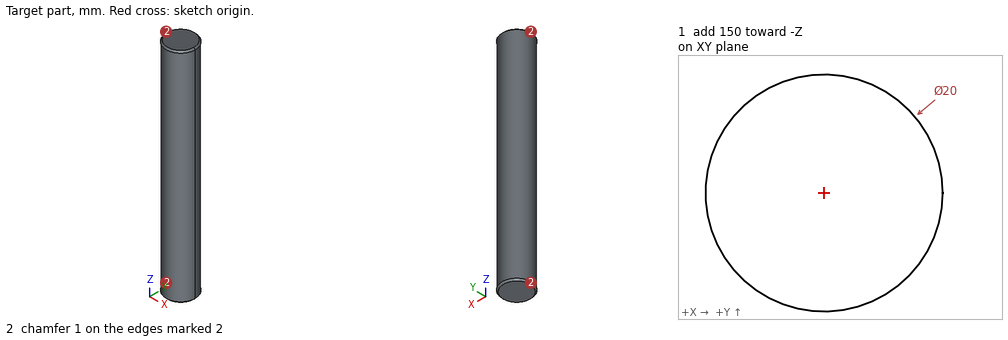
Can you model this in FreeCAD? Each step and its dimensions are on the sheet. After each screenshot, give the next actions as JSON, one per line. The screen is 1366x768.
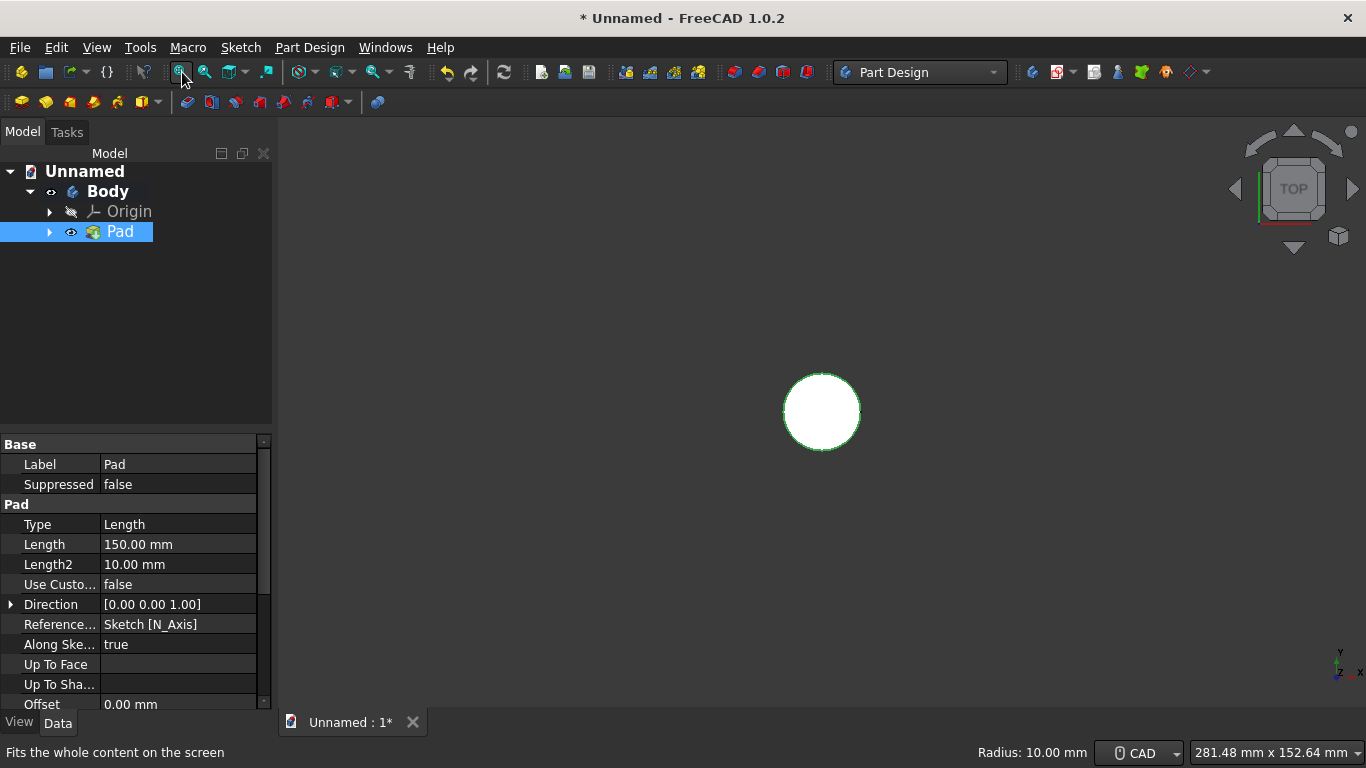
{"action": "key", "text": "1"}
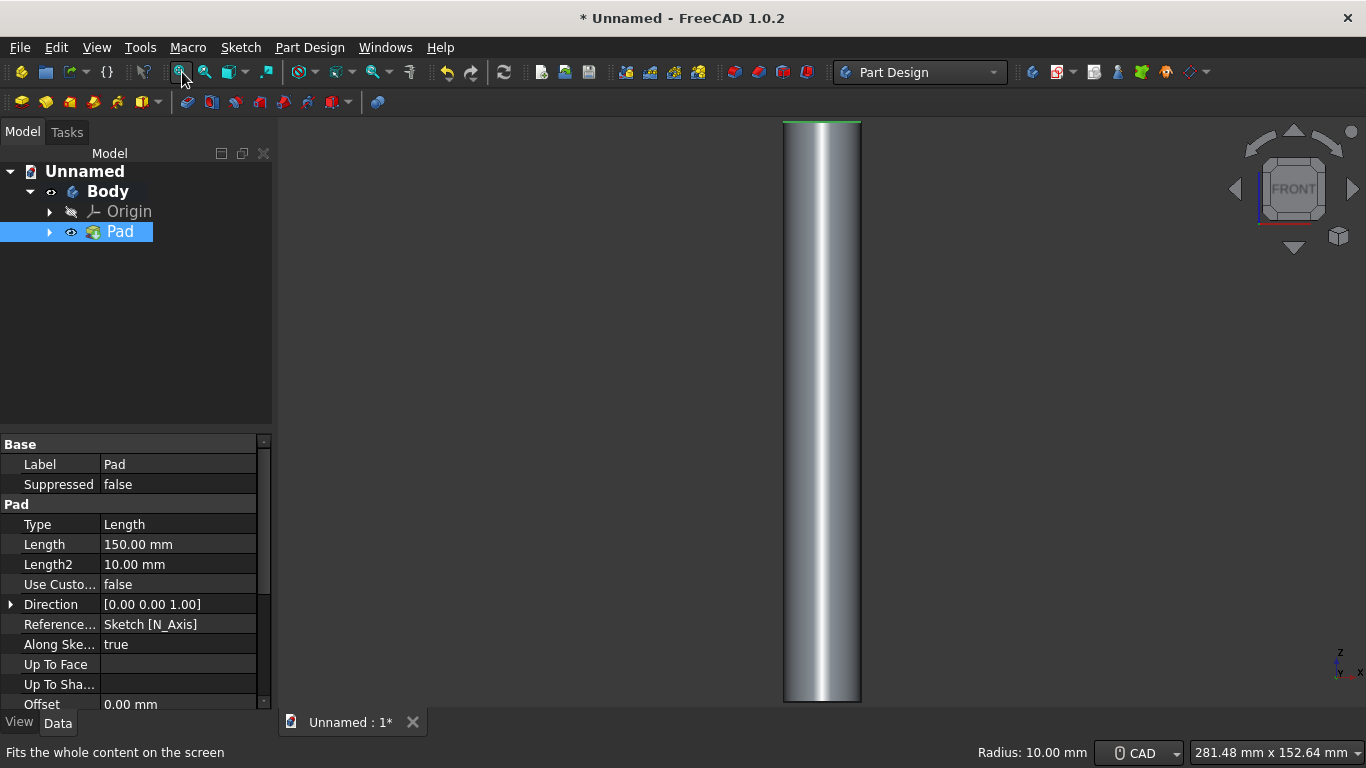
{"action": "key", "text": "3"}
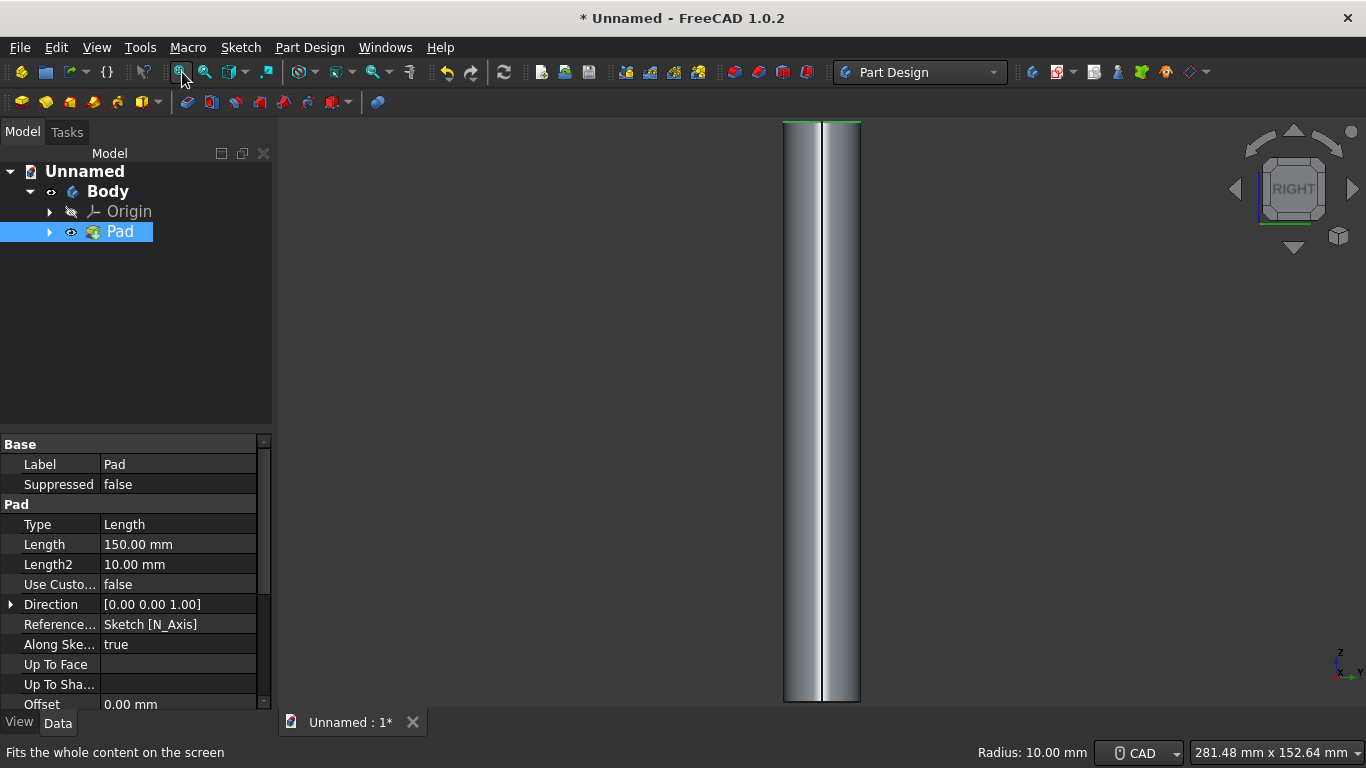
{"action": "key", "text": "5"}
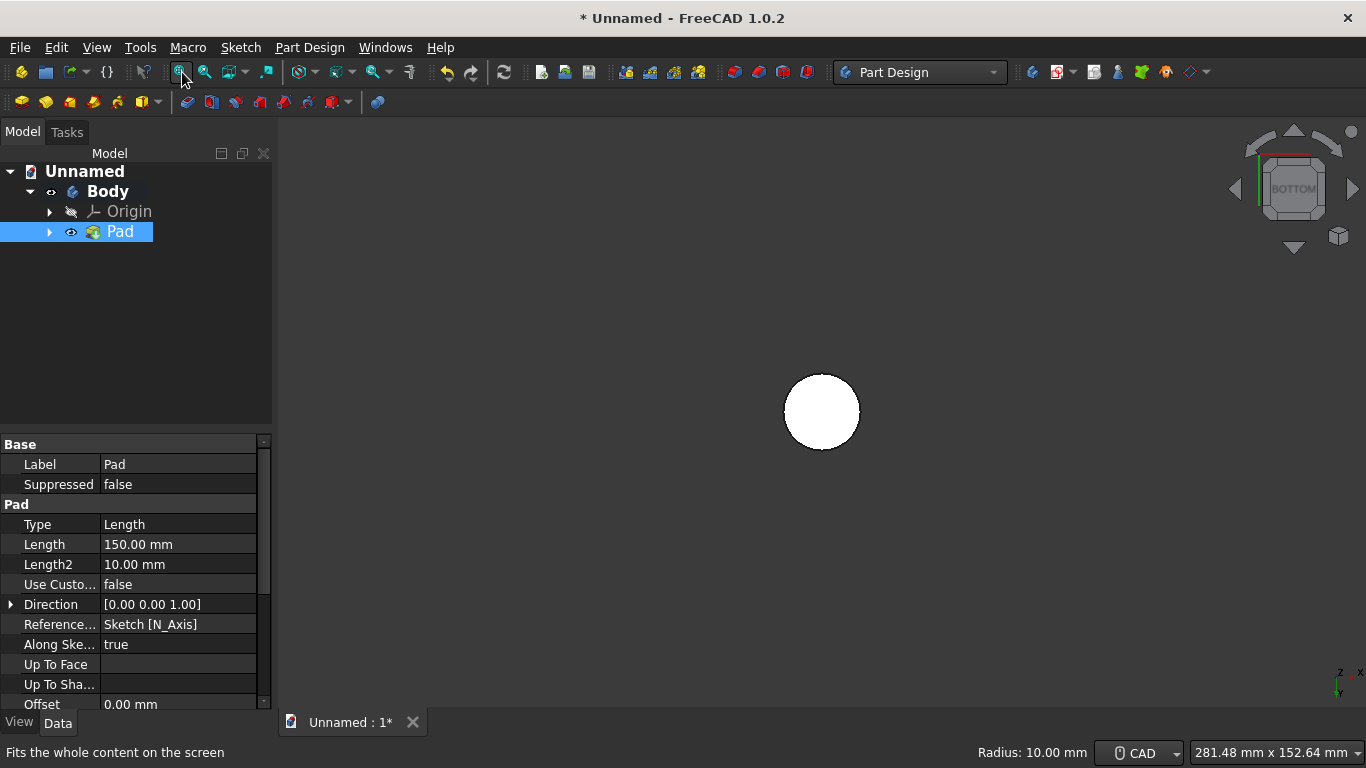
{"action": "key", "text": "v f"}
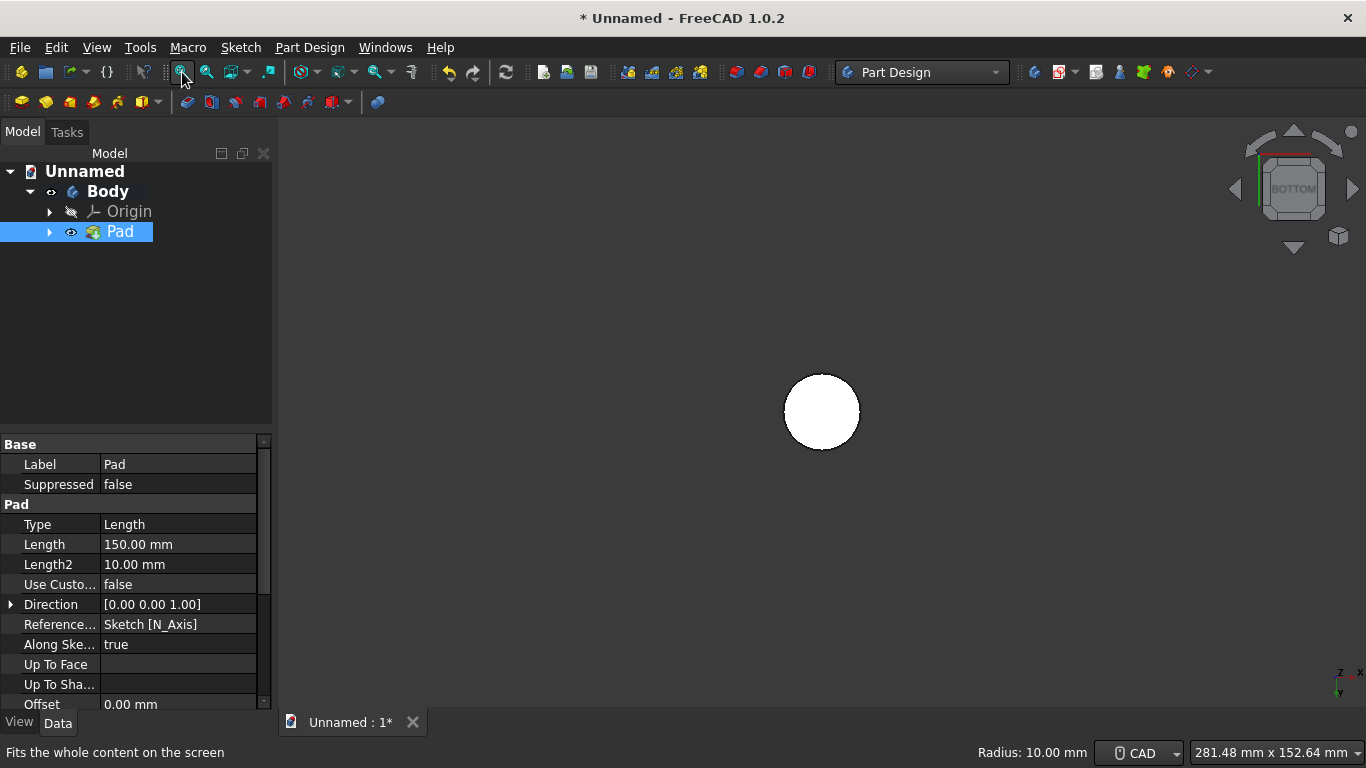
{"action": "left_click", "coordinate": [783, 411], "text": "ctrl"}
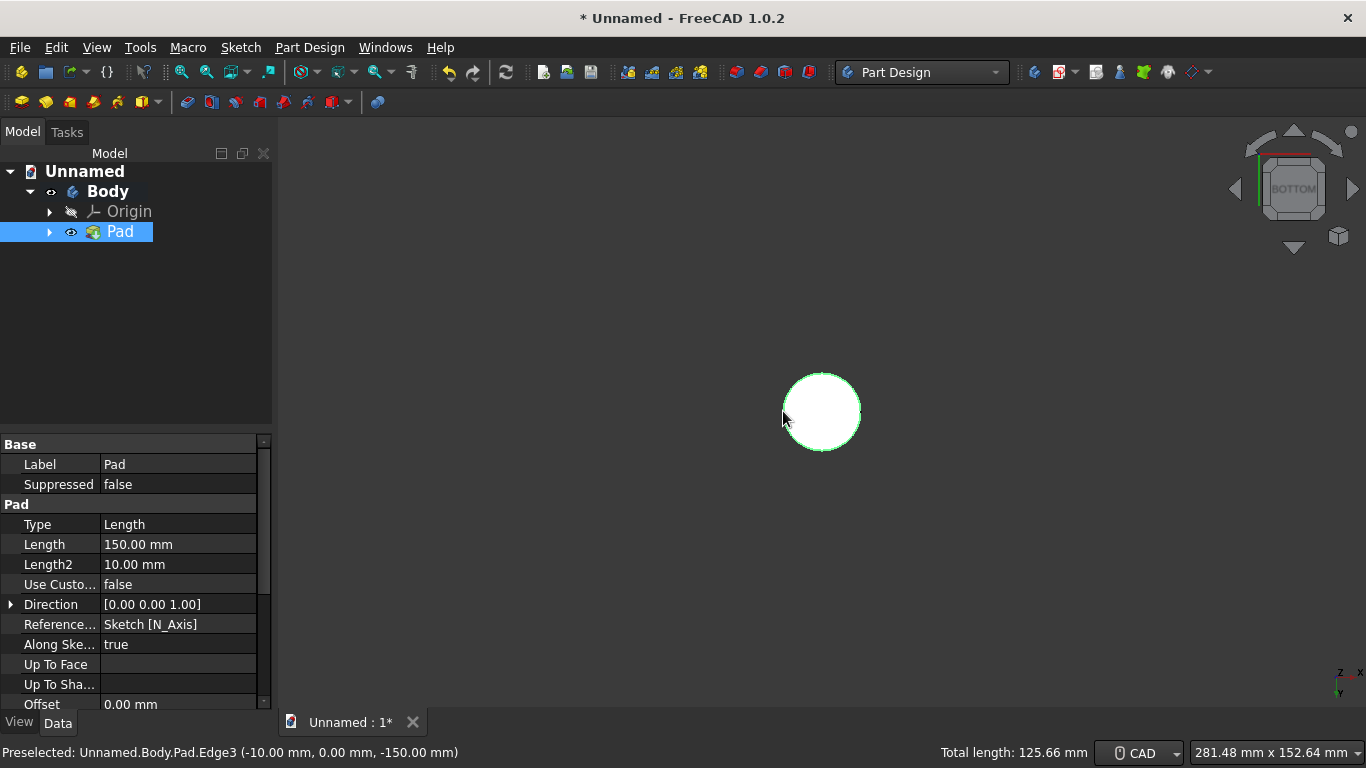
{"action": "left_click", "coordinate": [762, 72]}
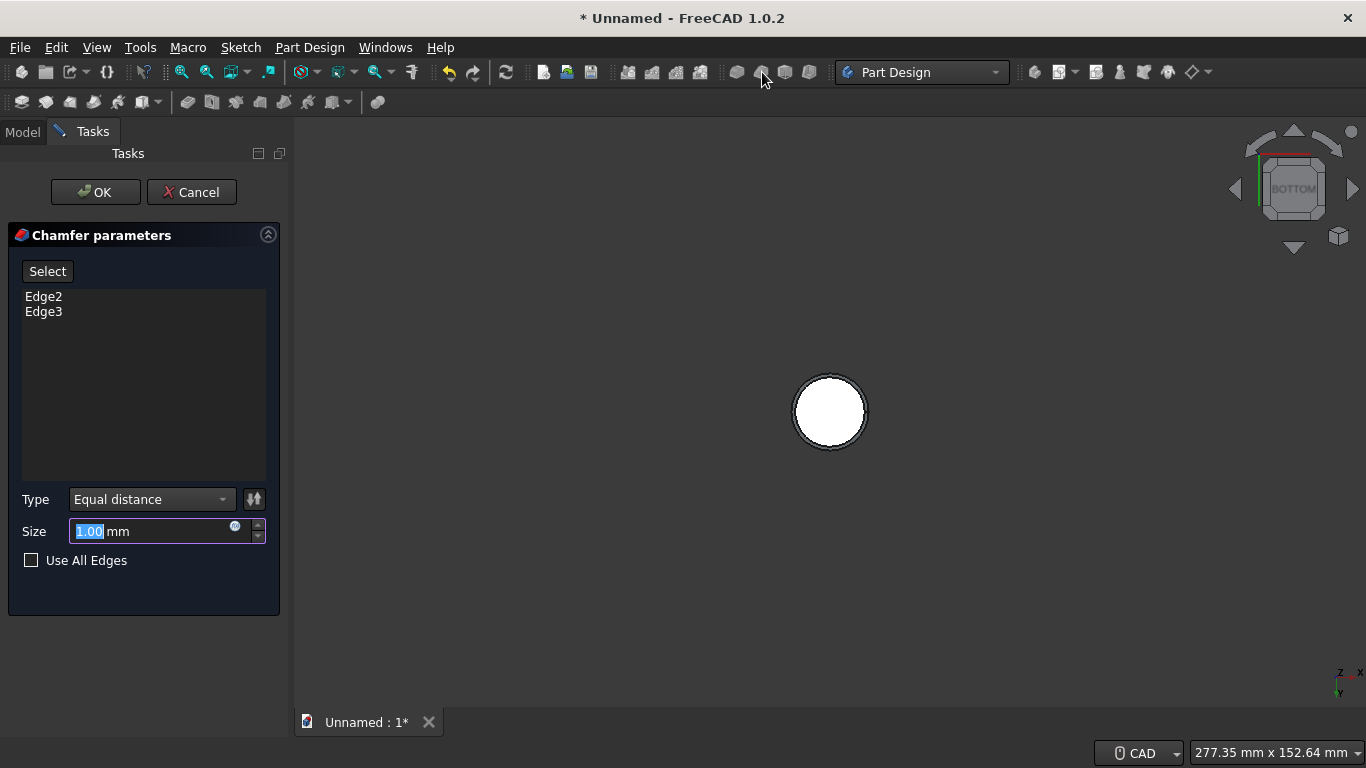
{"action": "type", "text": "1"}
{"action": "key", "text": "Tab"}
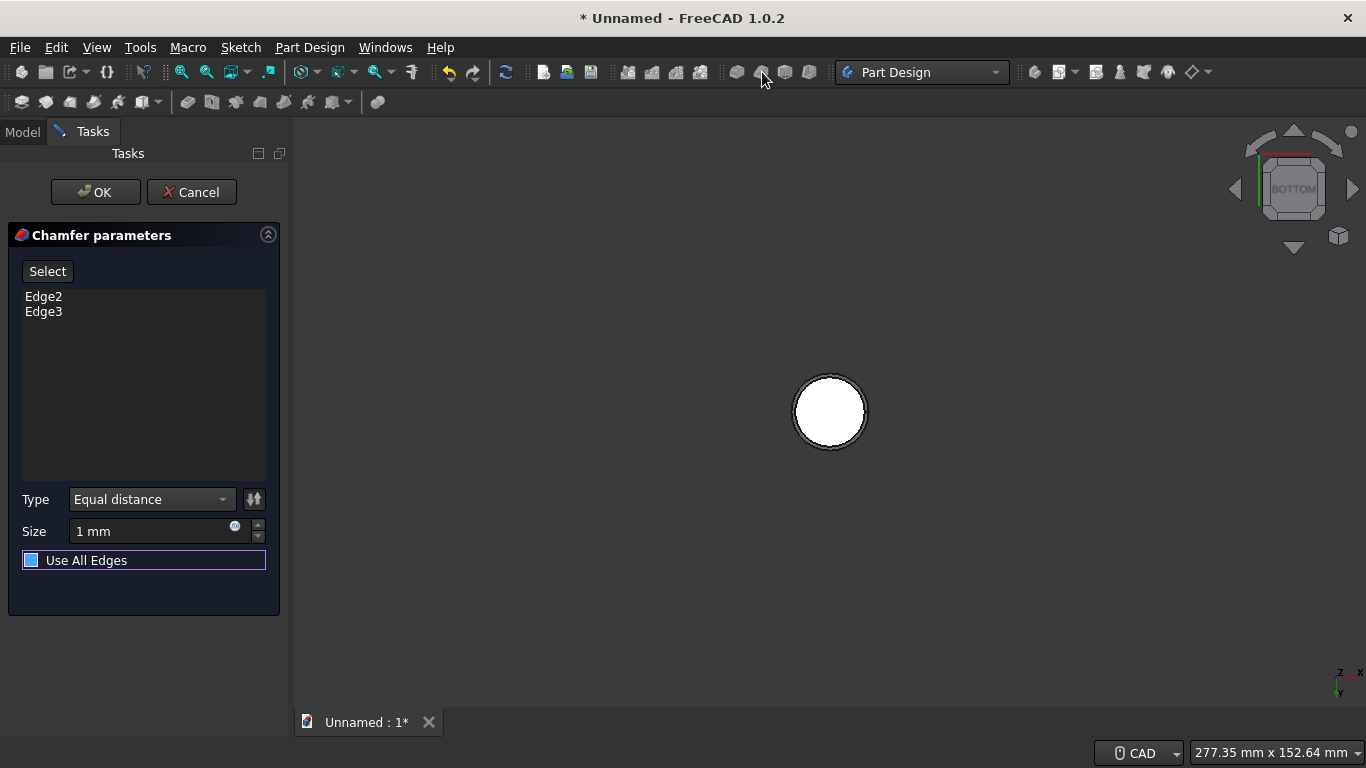
{"action": "left_click", "coordinate": [96, 192]}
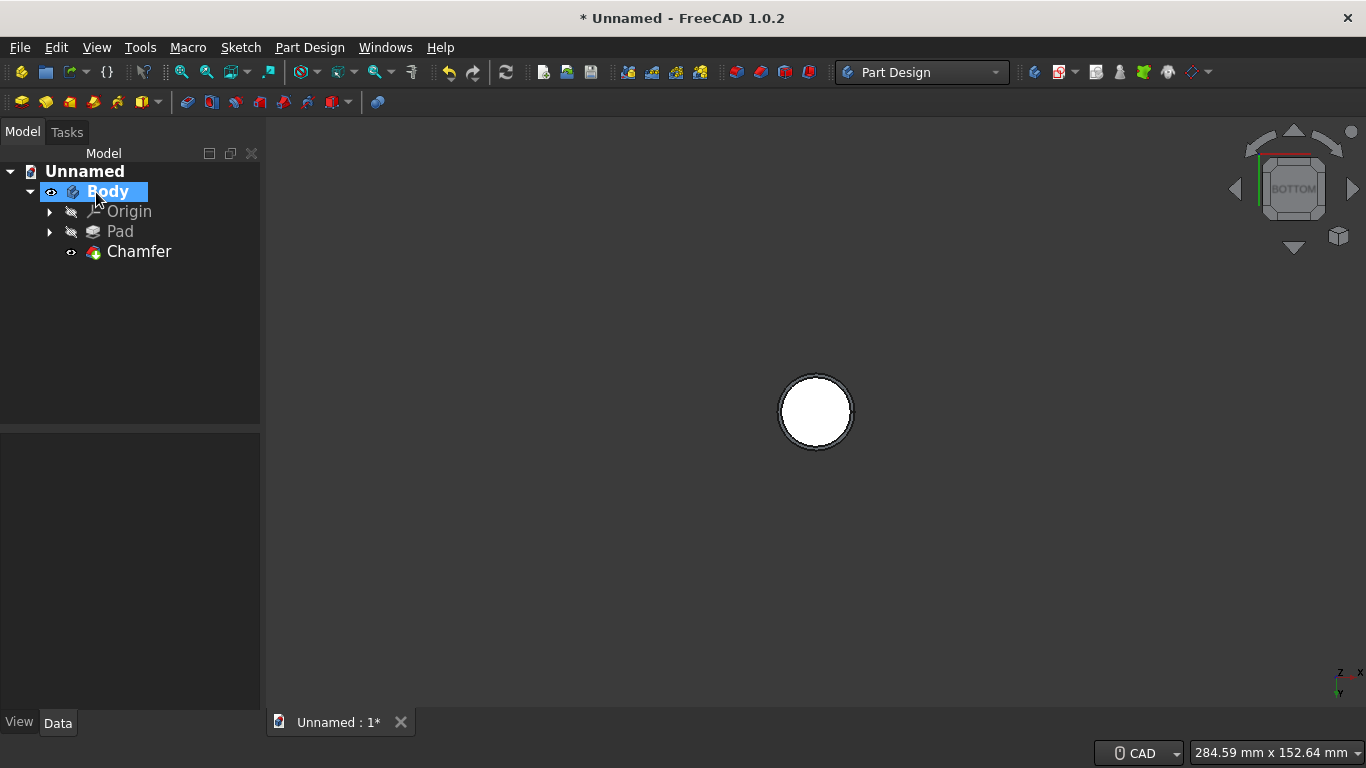
{"action": "key", "text": "0"}